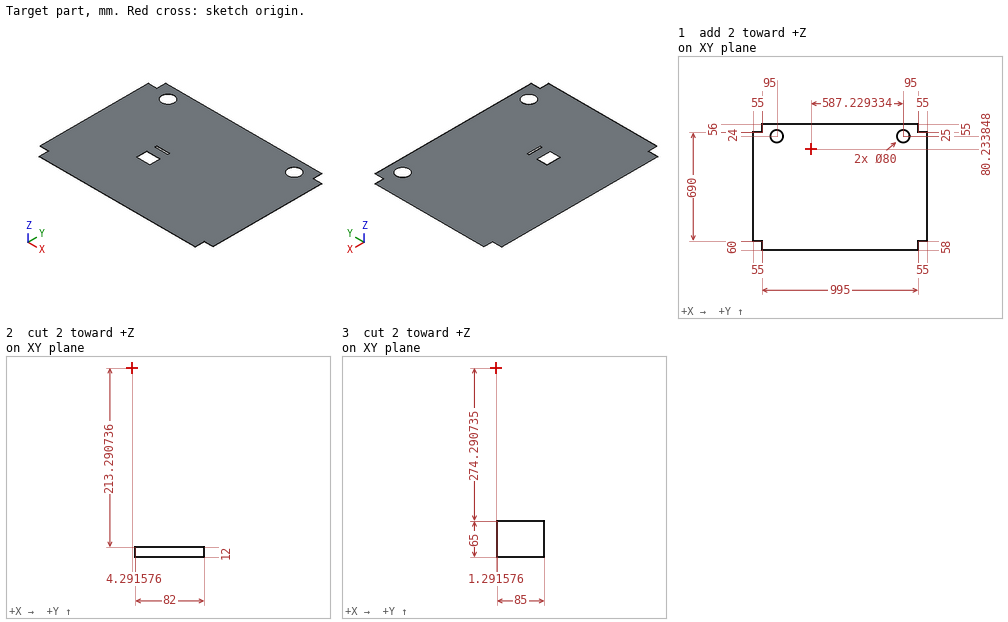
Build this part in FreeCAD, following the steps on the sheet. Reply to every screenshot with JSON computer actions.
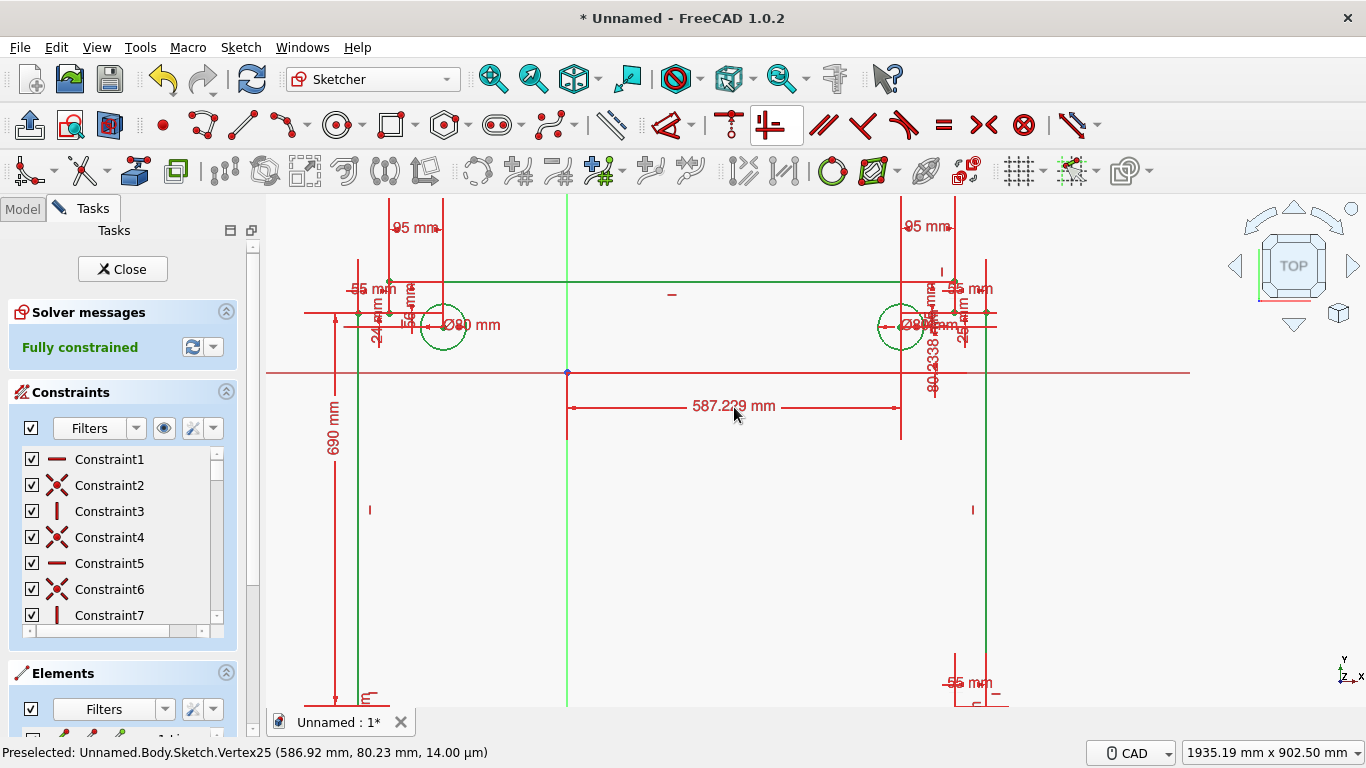
{"action": "left_click", "coordinate": [123, 269]}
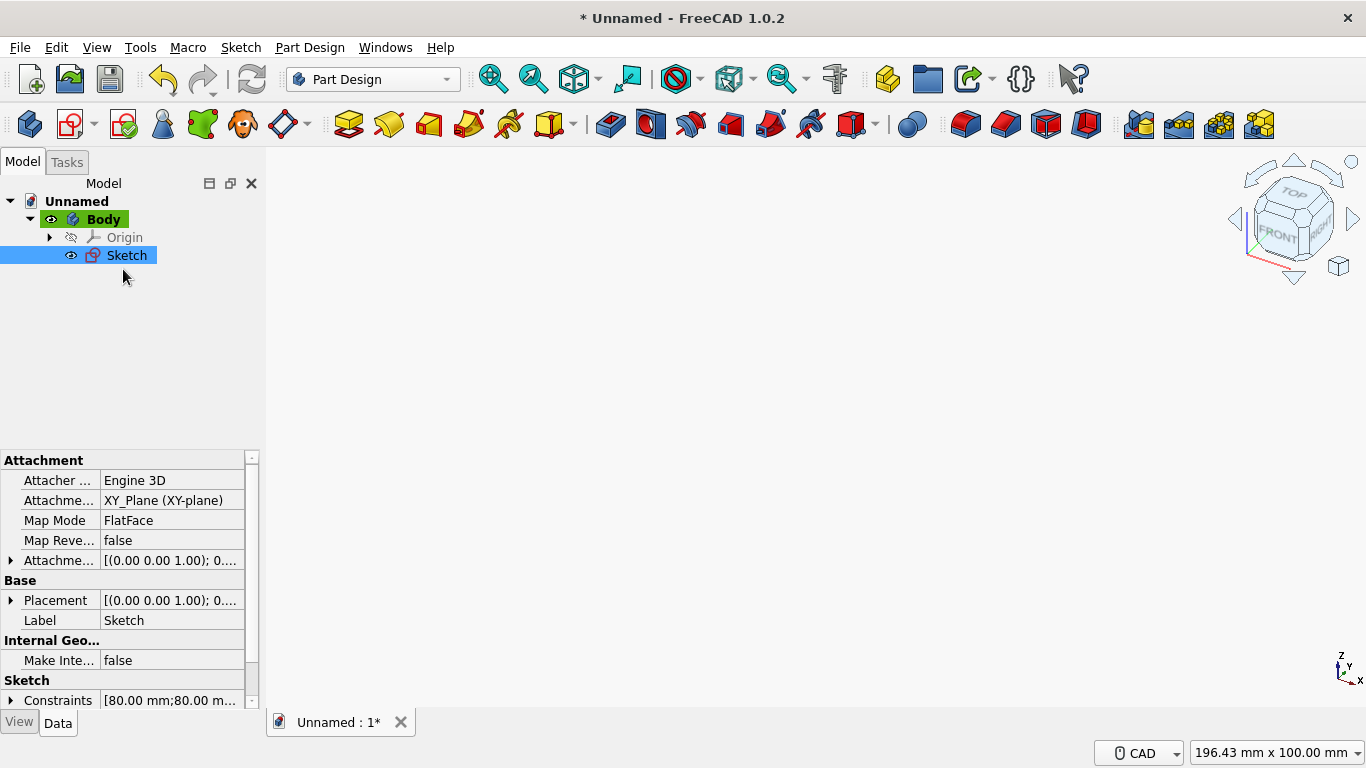
{"action": "left_click", "coordinate": [350, 124]}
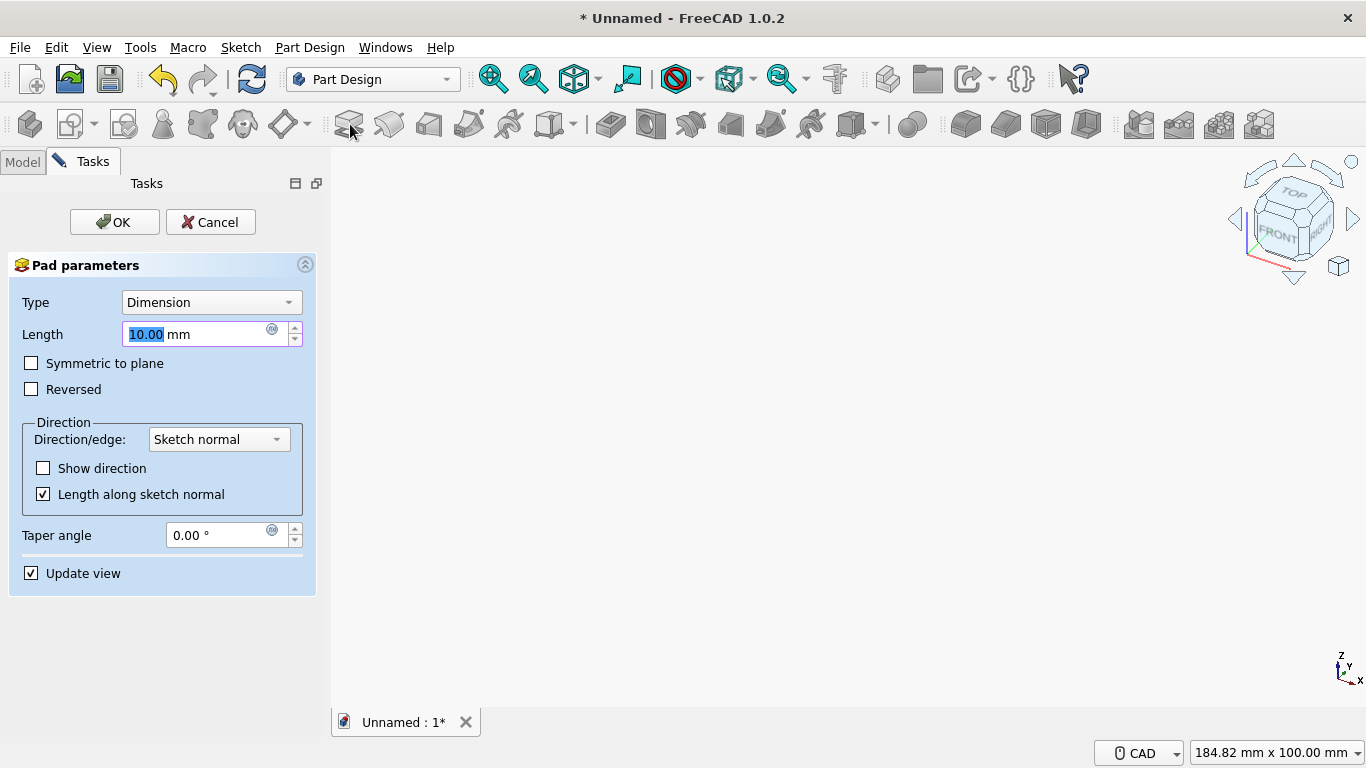
{"action": "type", "text": "2"}
{"action": "key", "text": "Tab"}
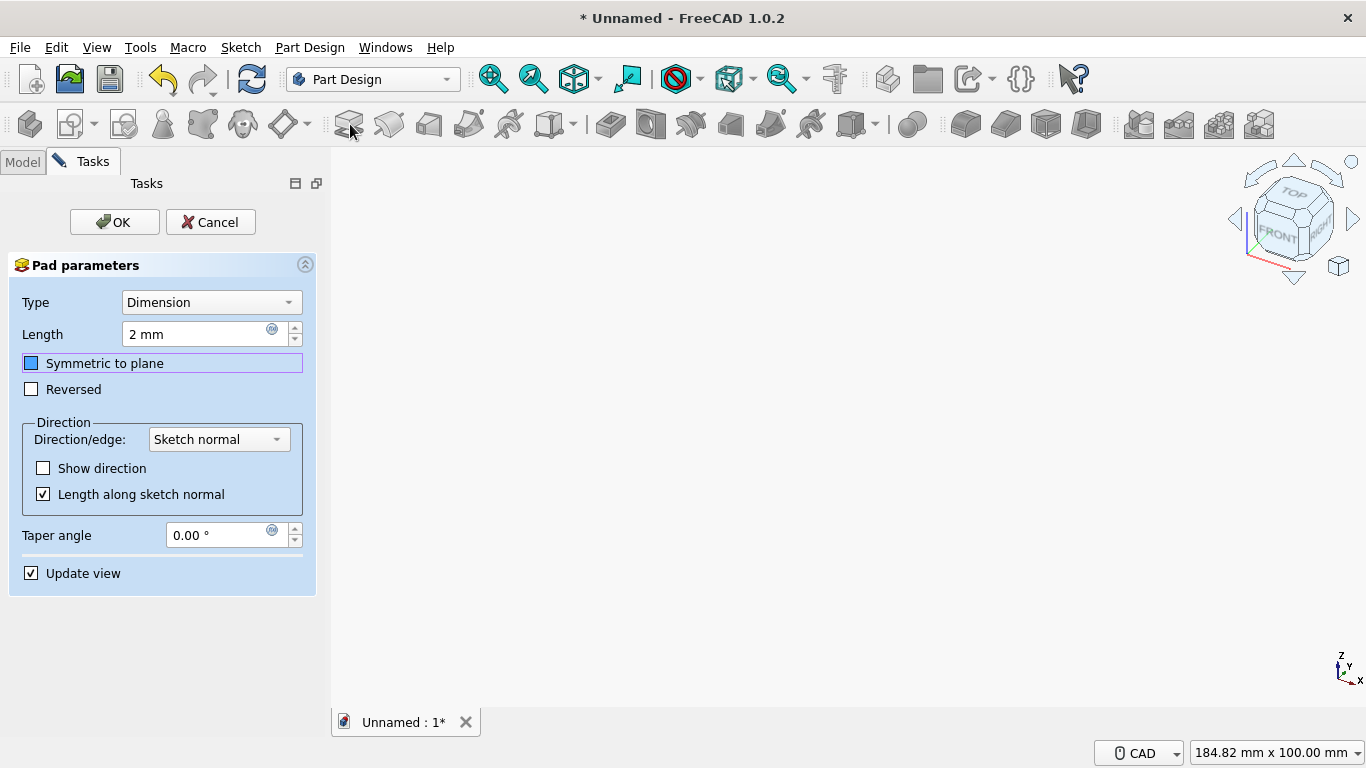
{"action": "left_click", "coordinate": [115, 222]}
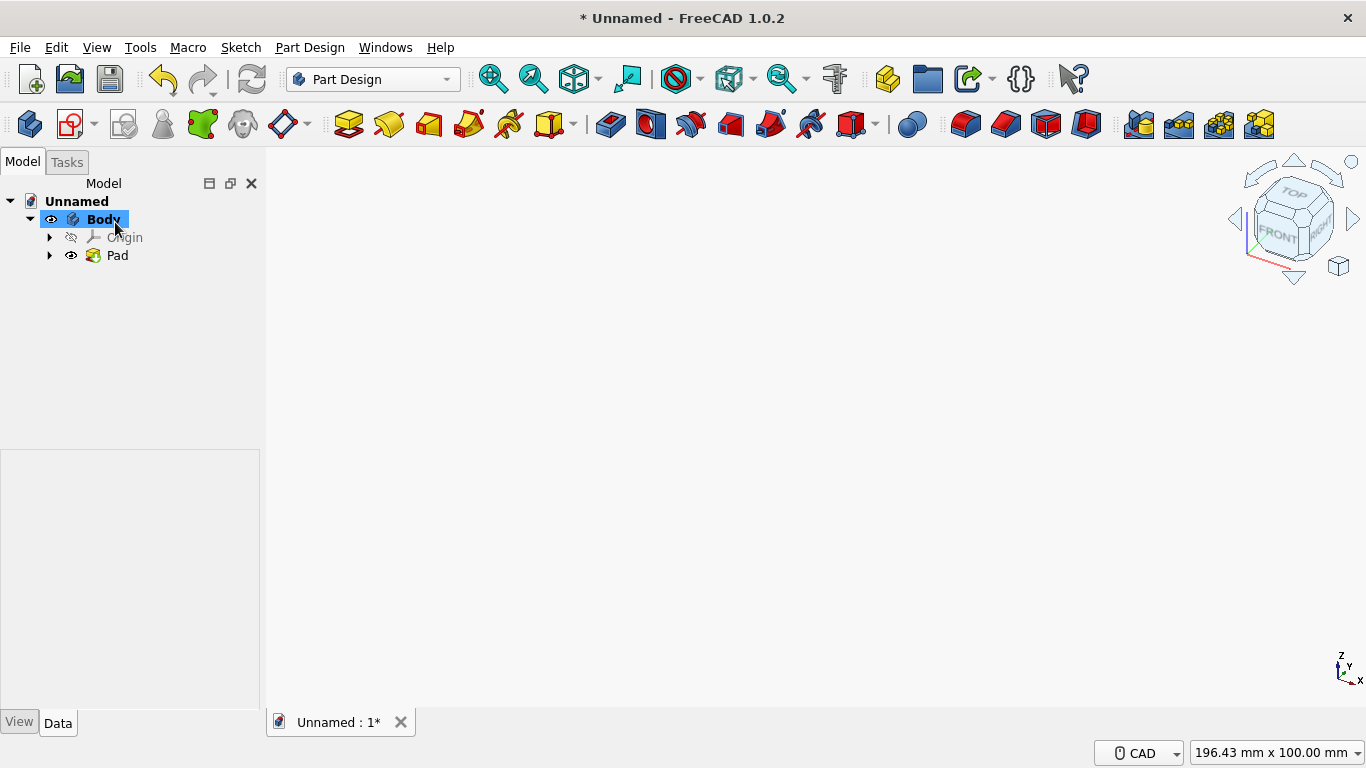
{"action": "left_click", "coordinate": [494, 80]}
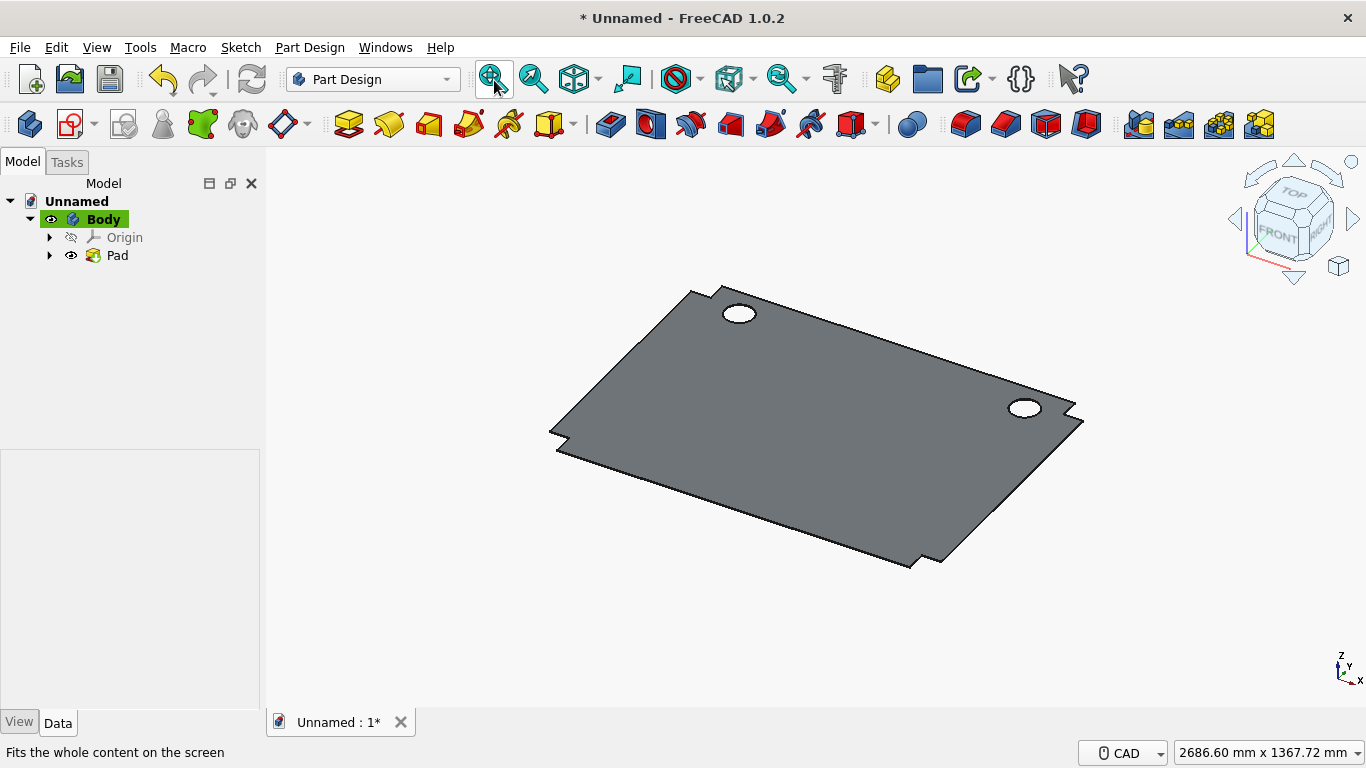
{"action": "left_click", "coordinate": [70, 124]}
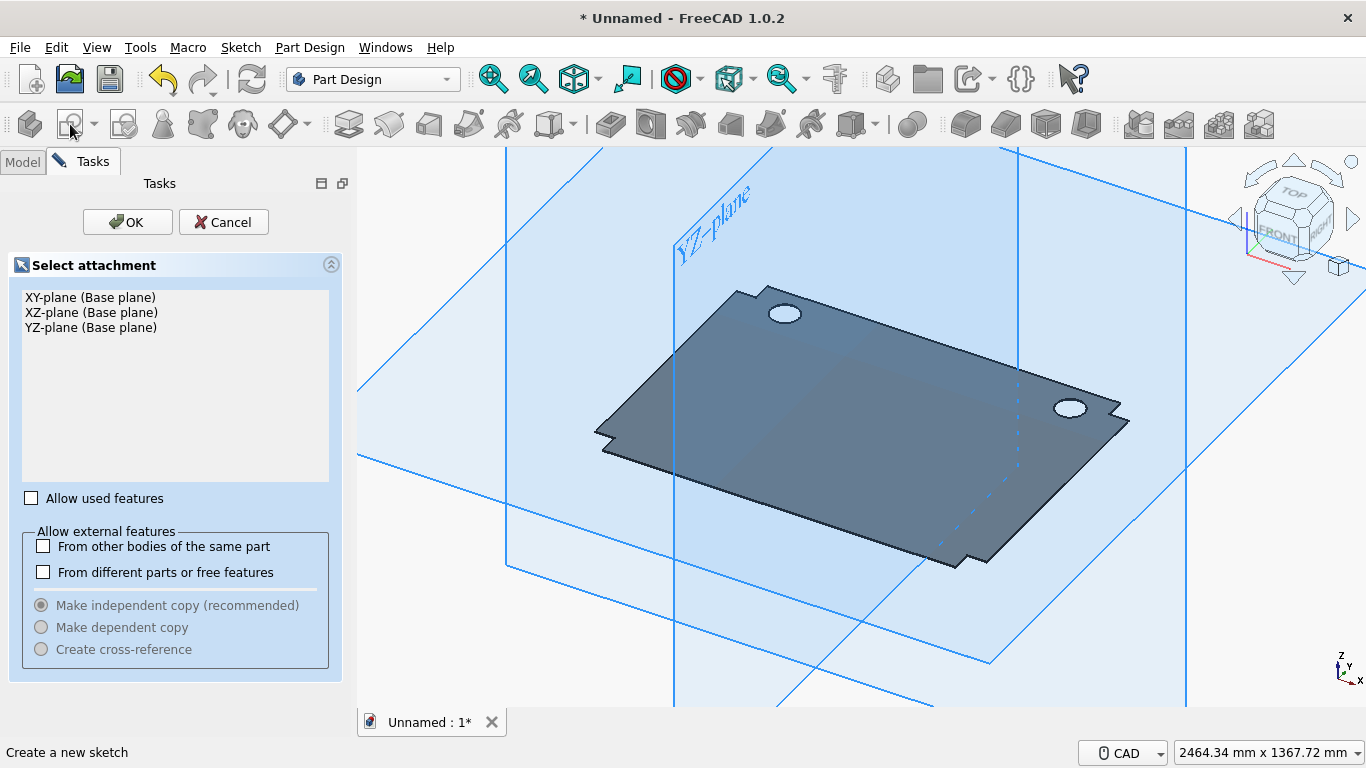
{"action": "left_click", "coordinate": [82, 298]}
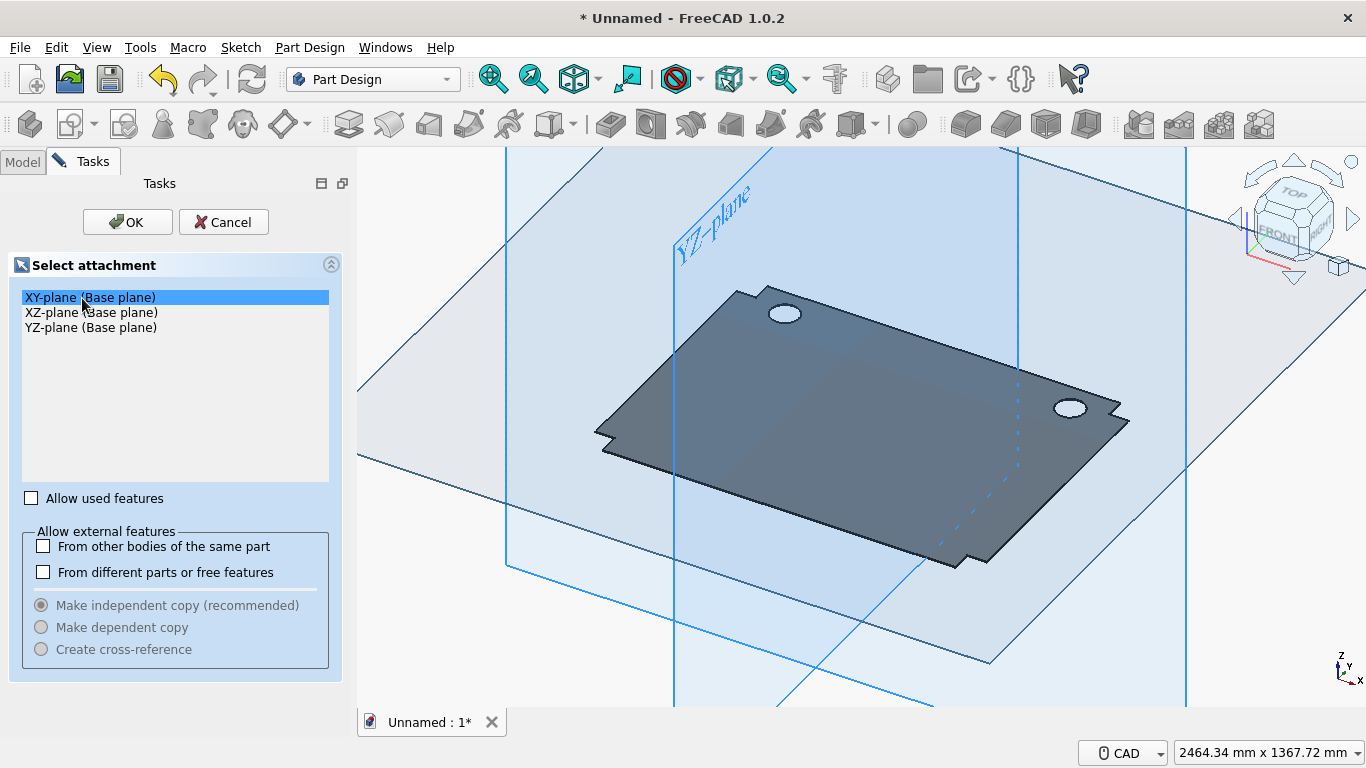
{"action": "left_click", "coordinate": [128, 222]}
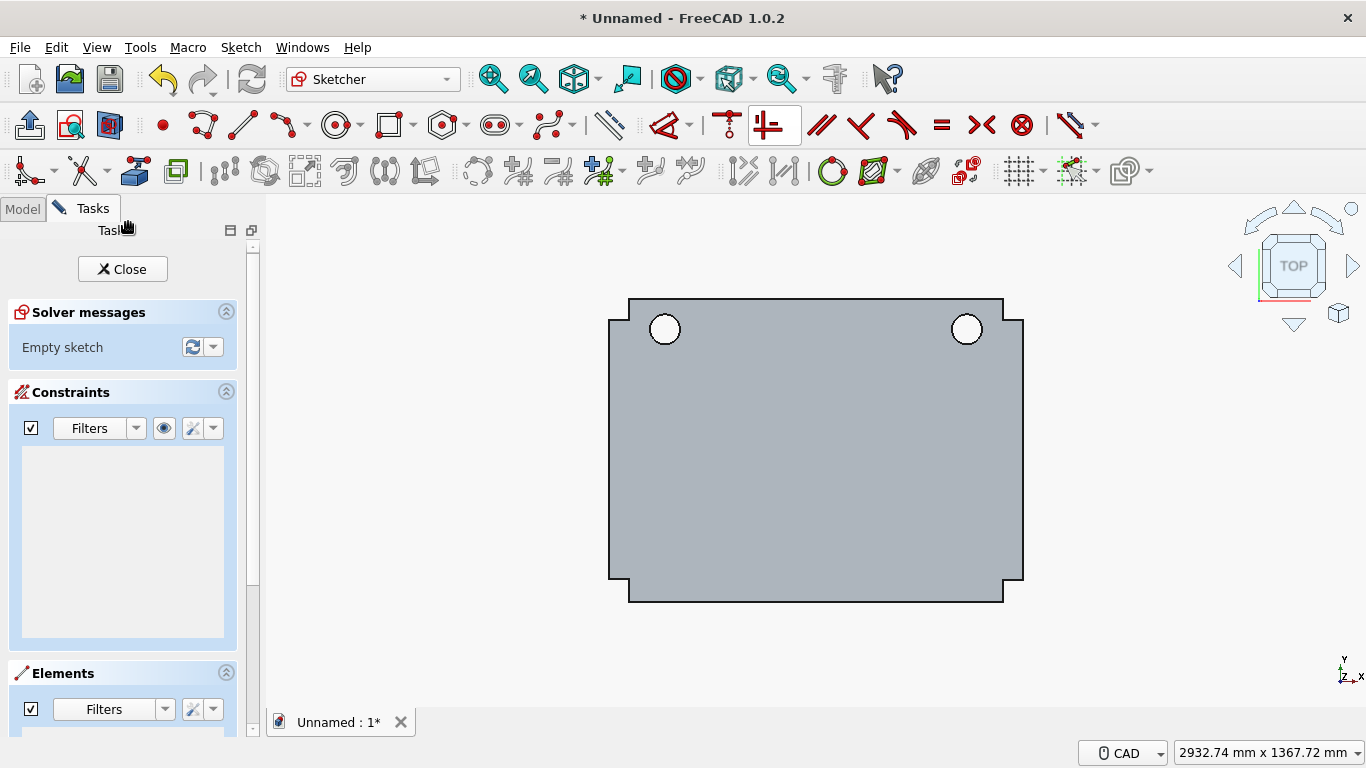
{"action": "left_click", "coordinate": [110, 126]}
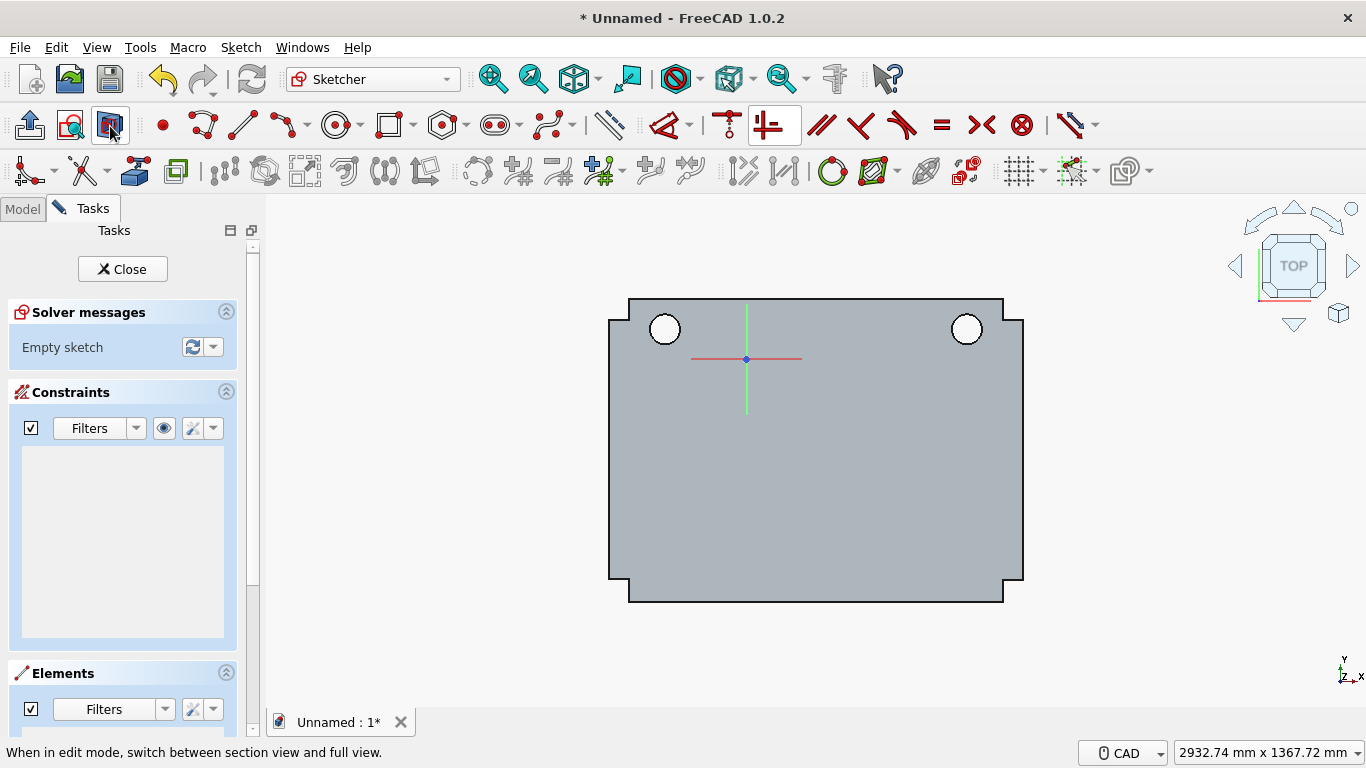
{"action": "scroll", "coordinate": [765, 441], "scroll_direction": "up", "scroll_amount": 15}